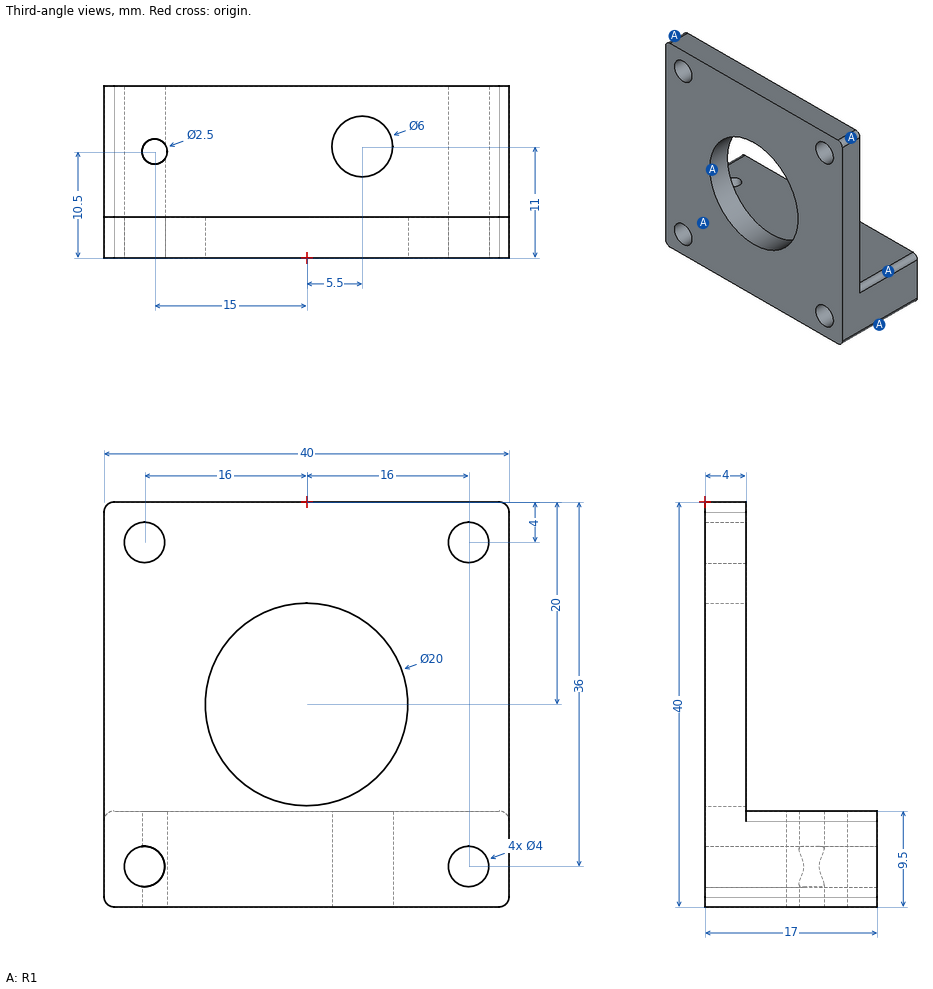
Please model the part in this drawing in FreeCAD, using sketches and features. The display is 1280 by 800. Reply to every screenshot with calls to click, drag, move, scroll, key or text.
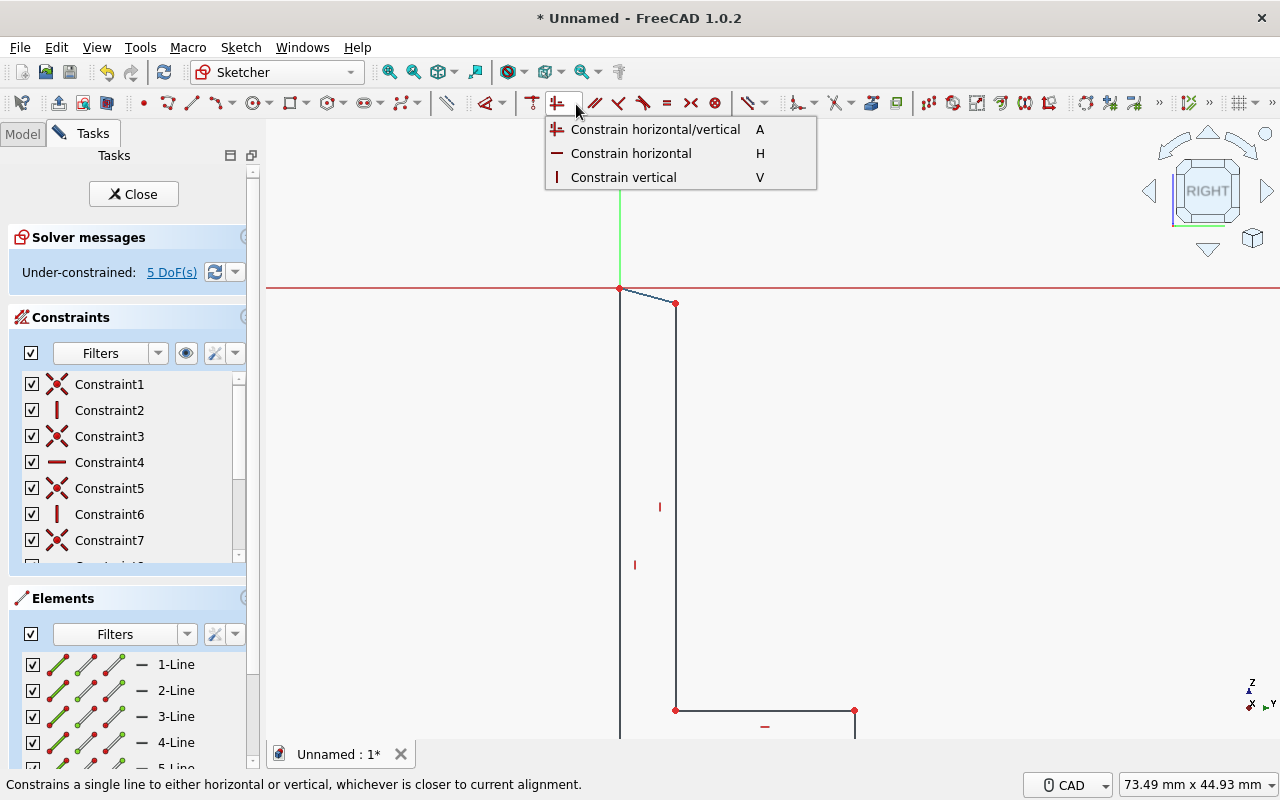
click(681, 153)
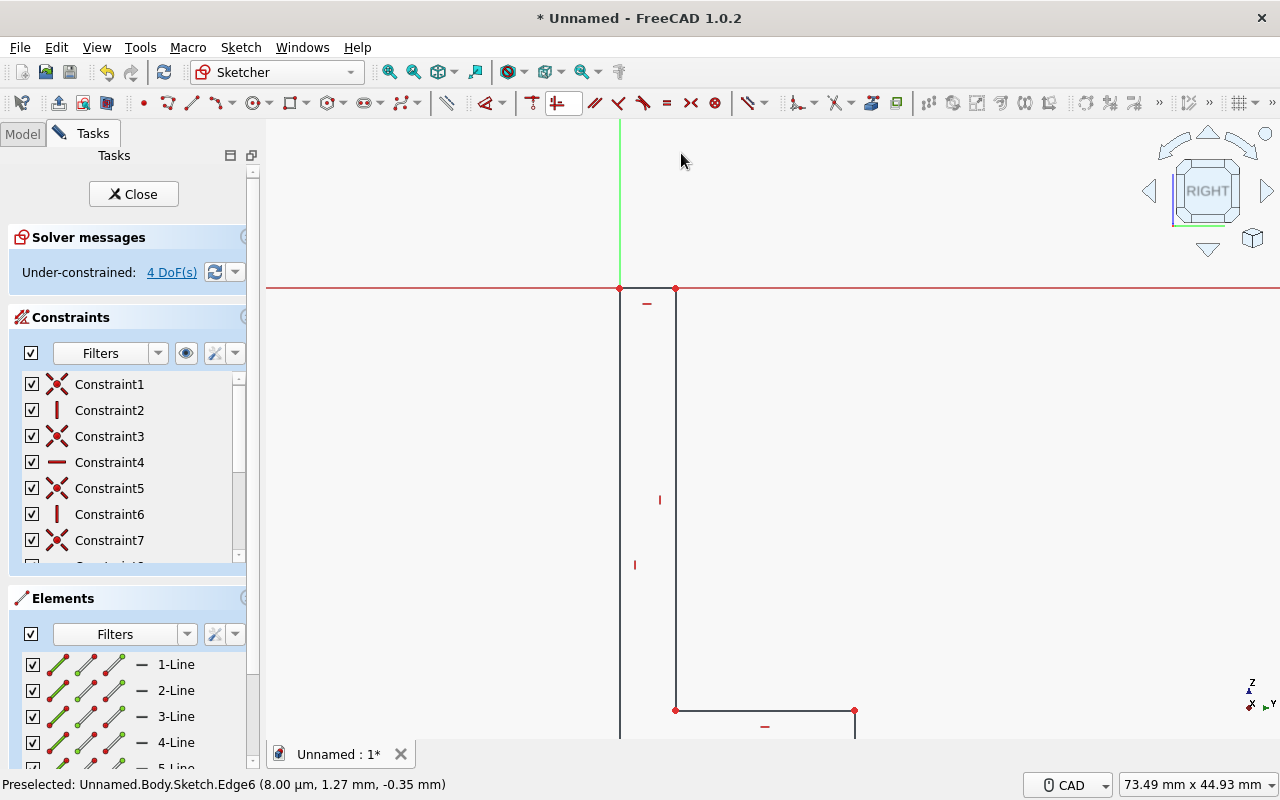
key(d)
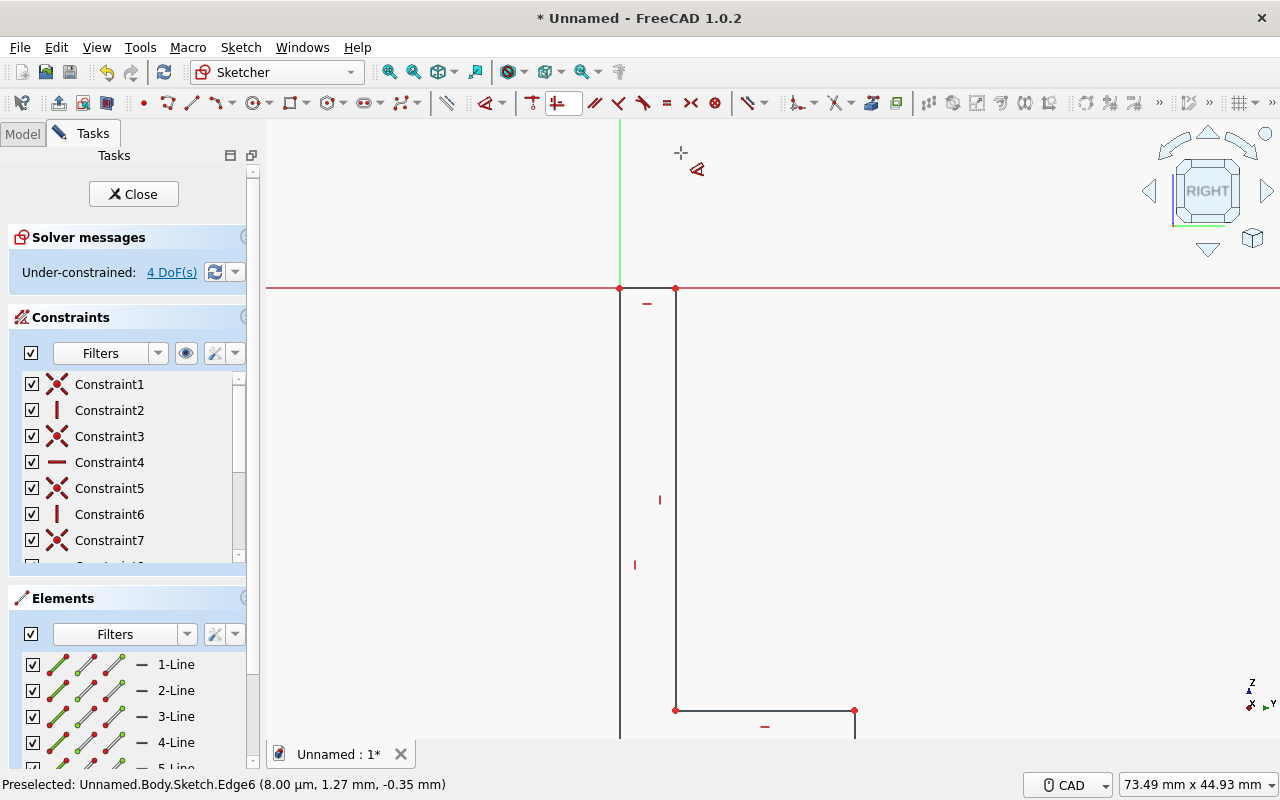
click(659, 288)
click(648, 254)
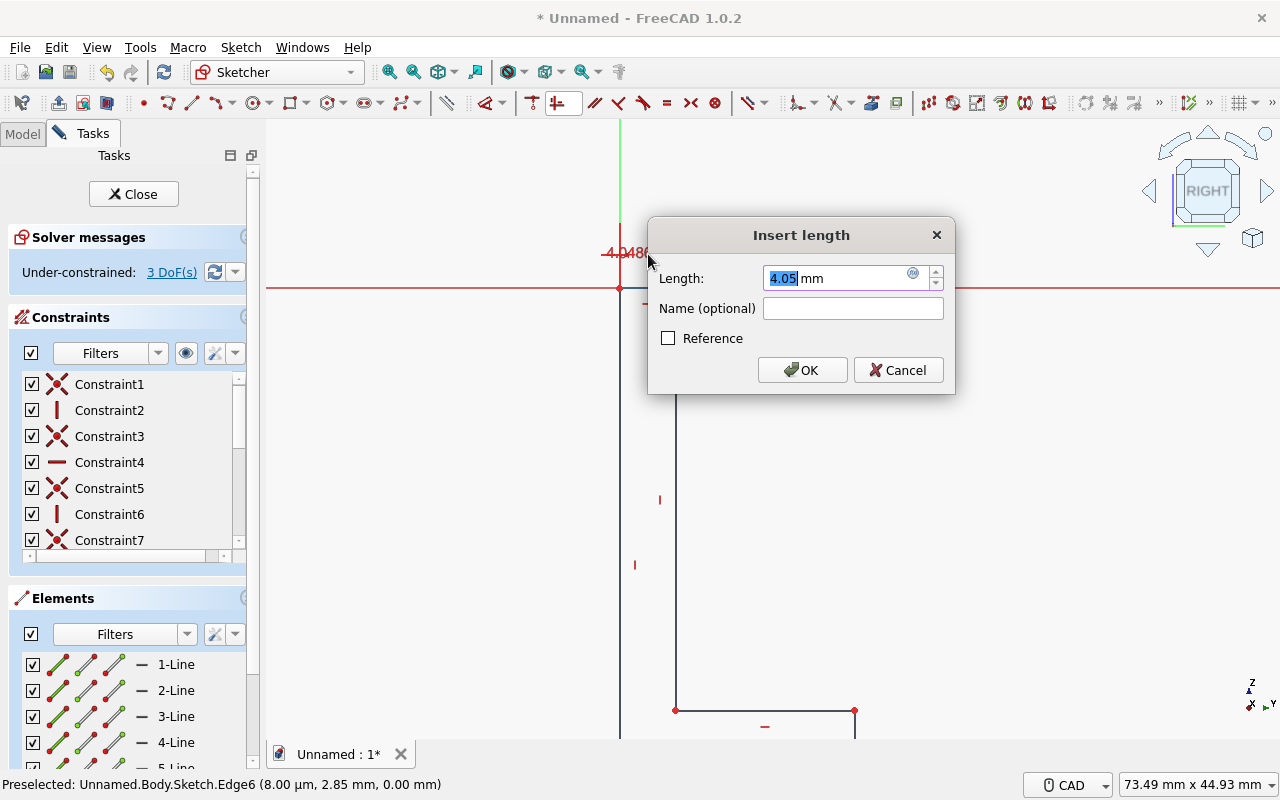
text(4)
key(Return)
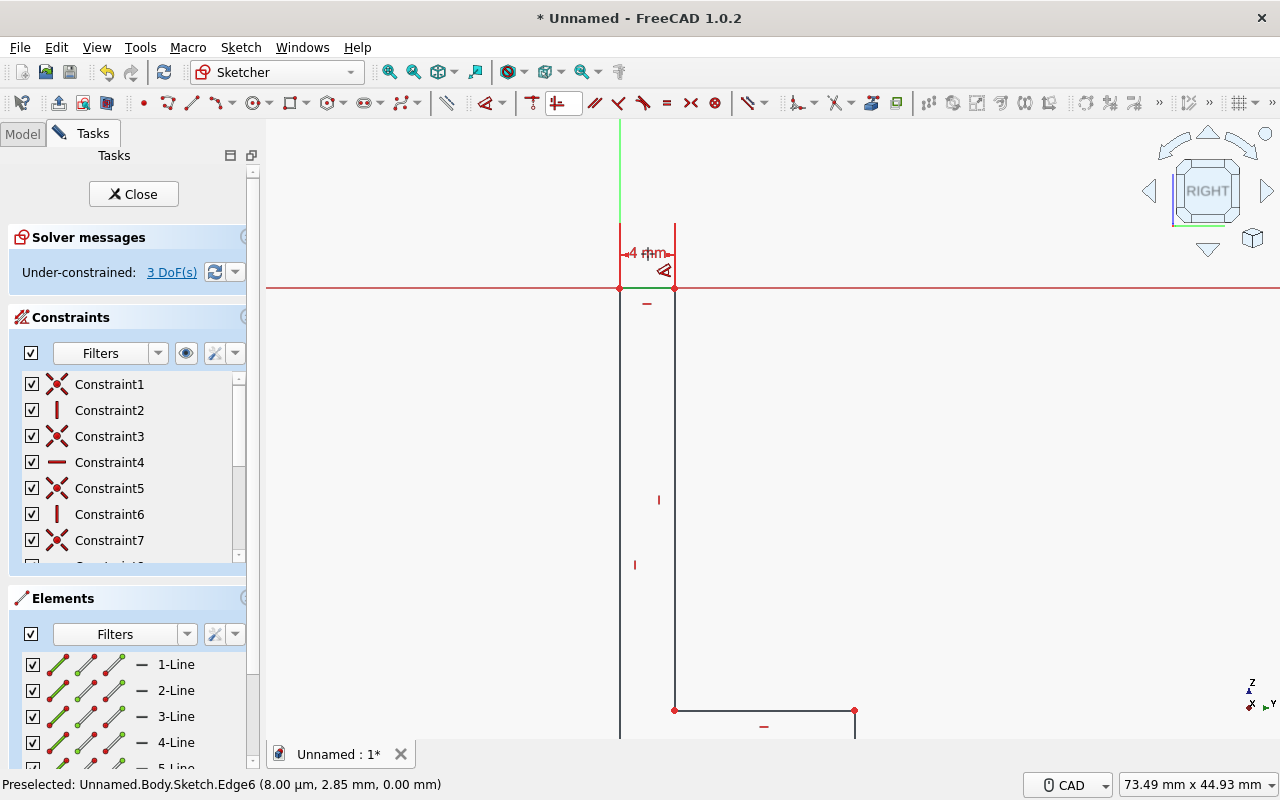
click(620, 454)
click(586, 500)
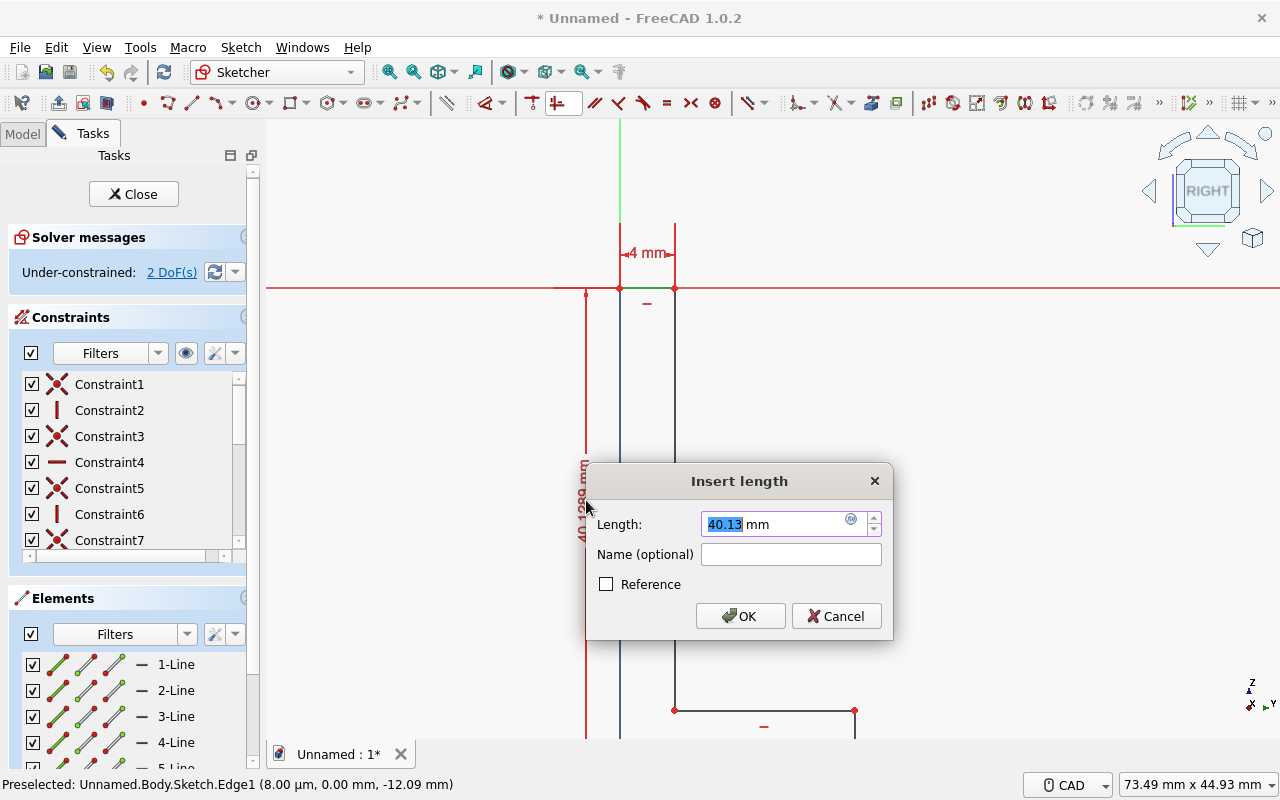
text(40)
key(Return)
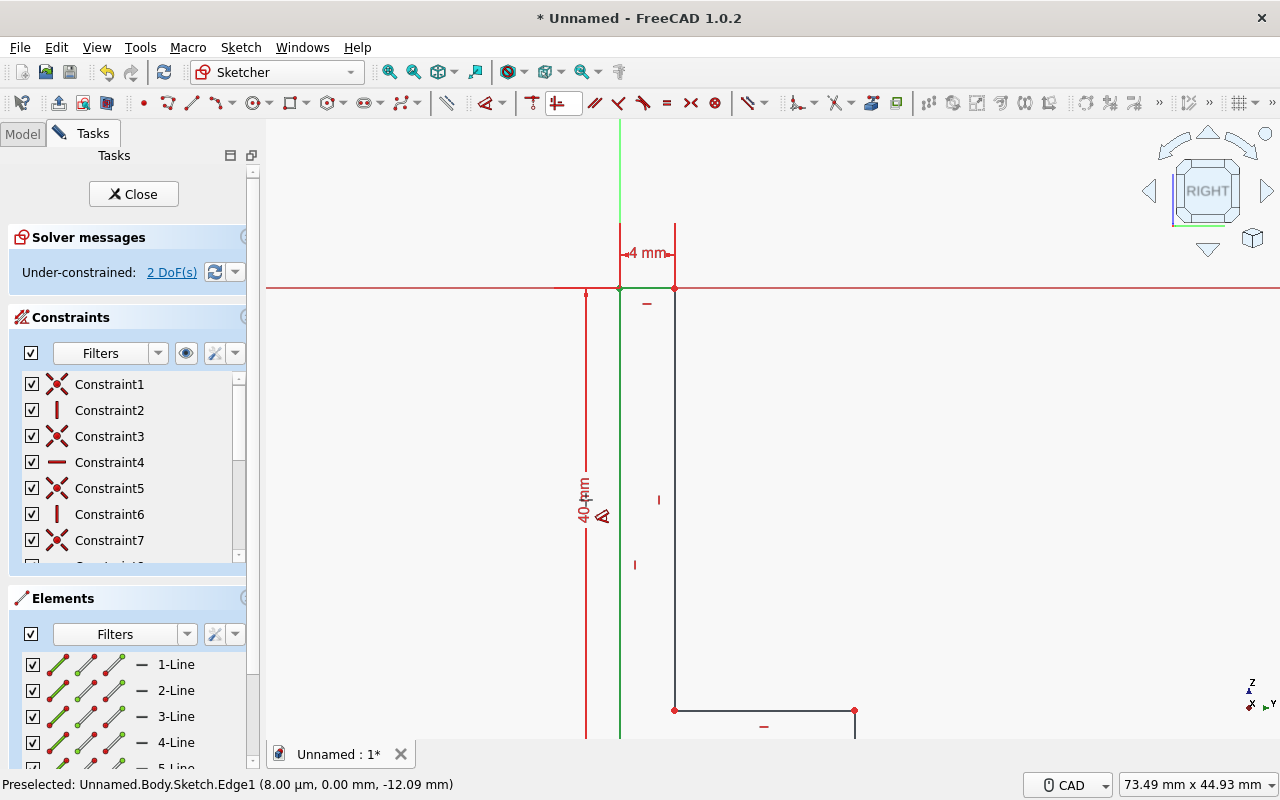
scroll(638, 154, down, 2)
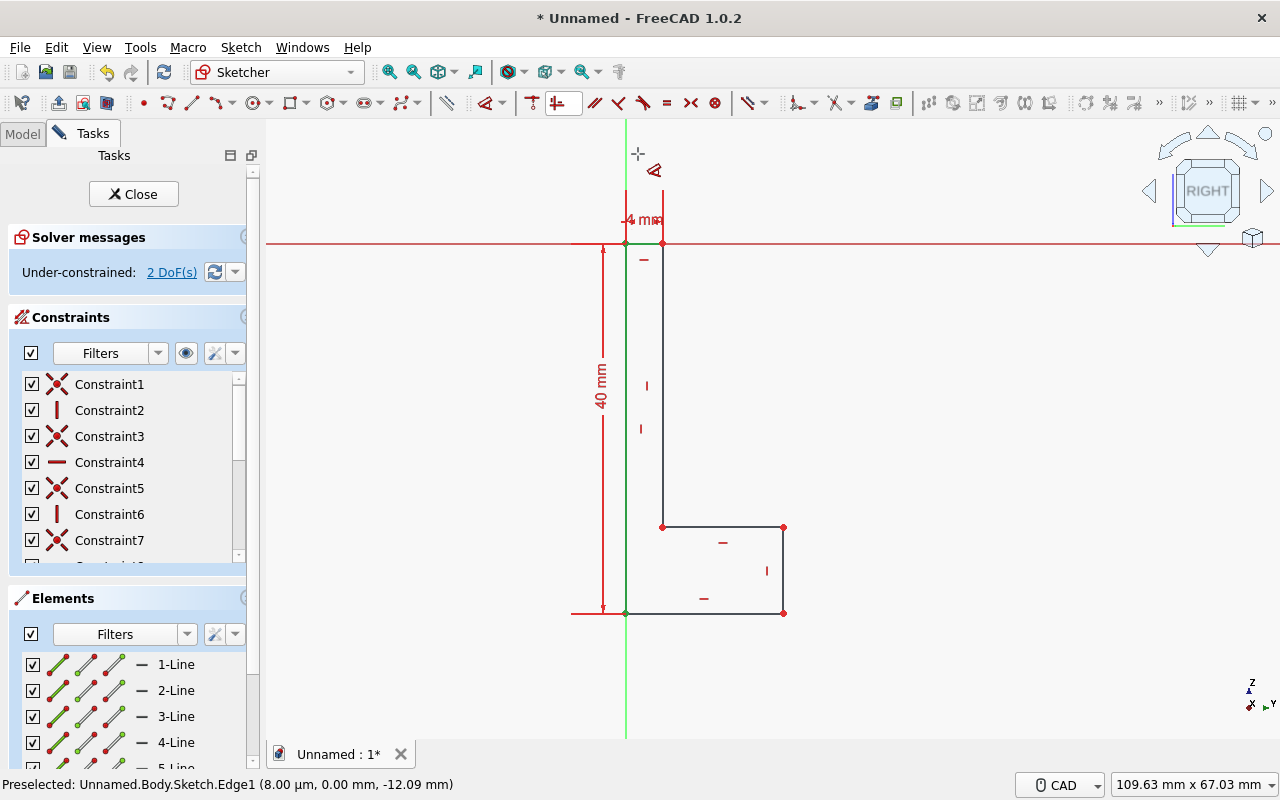
click(673, 614)
click(705, 648)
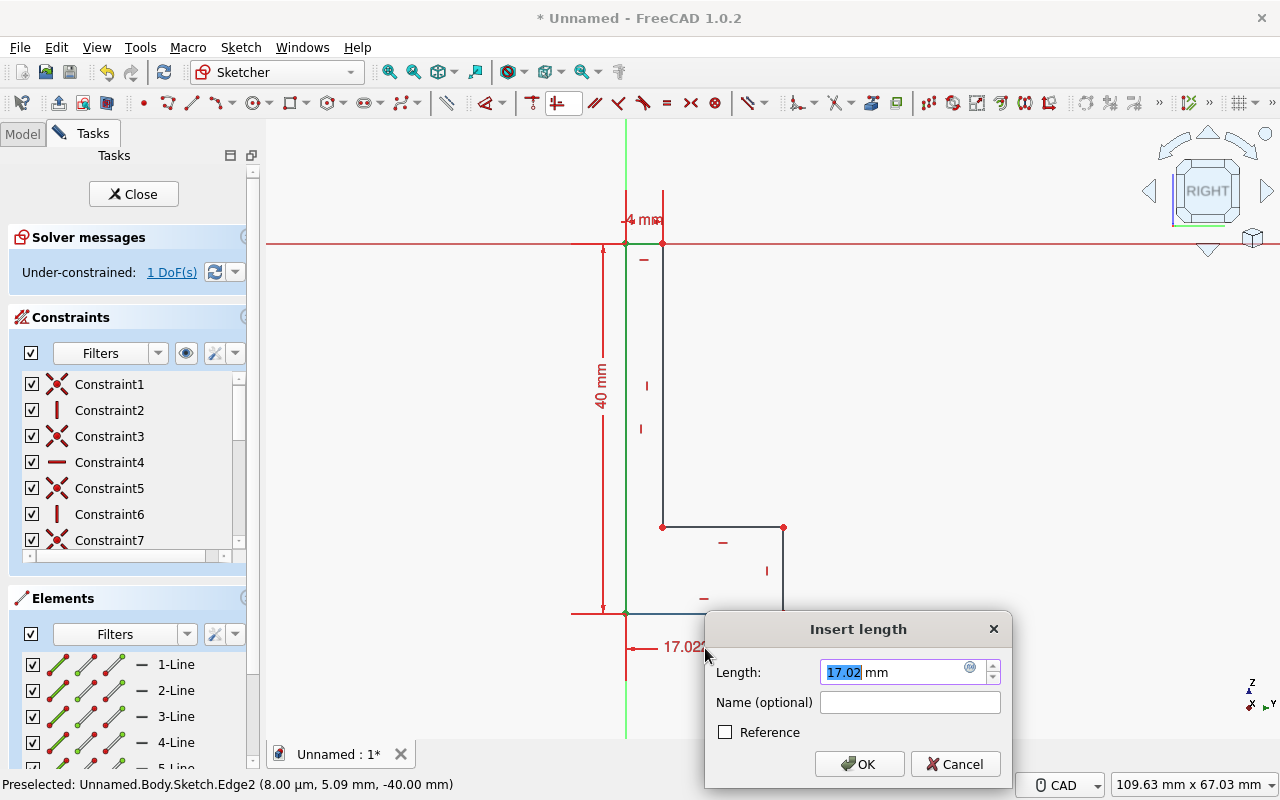
text(17)
key(Return)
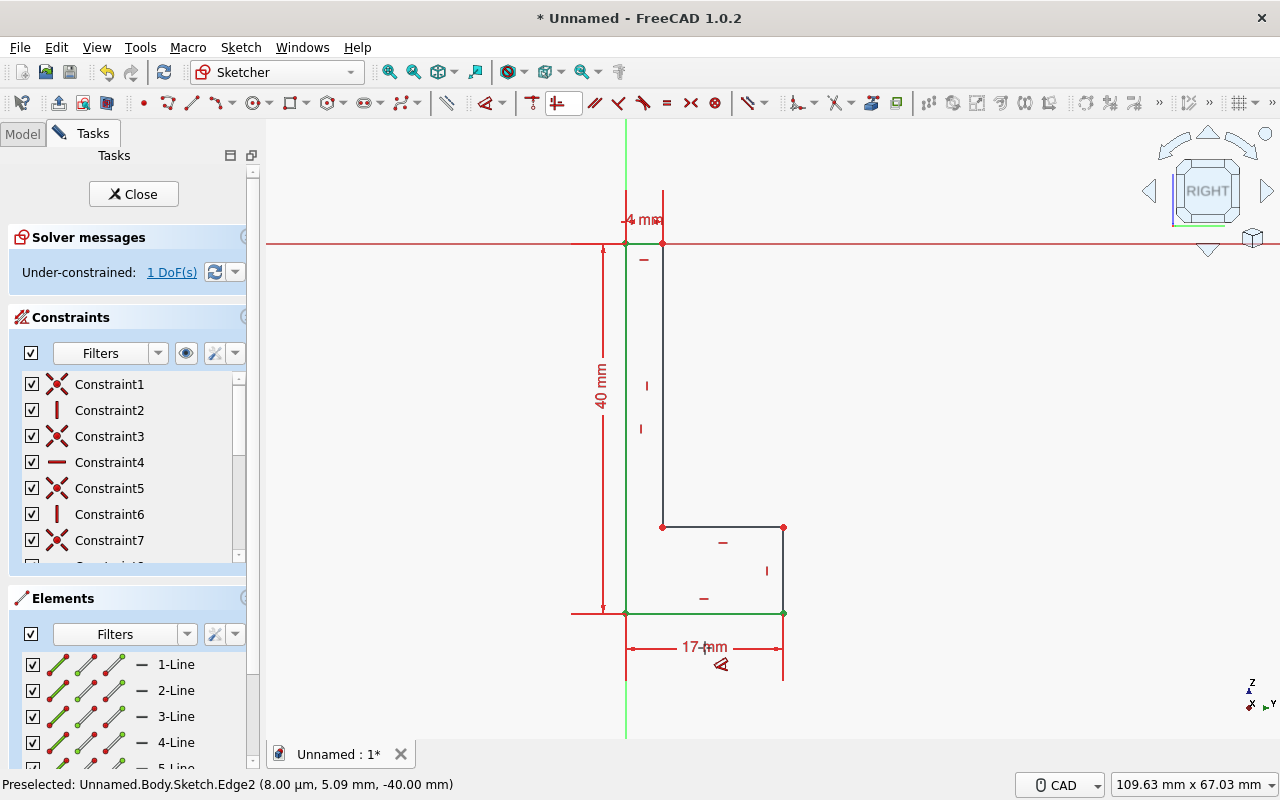
click(783, 588)
click(817, 571)